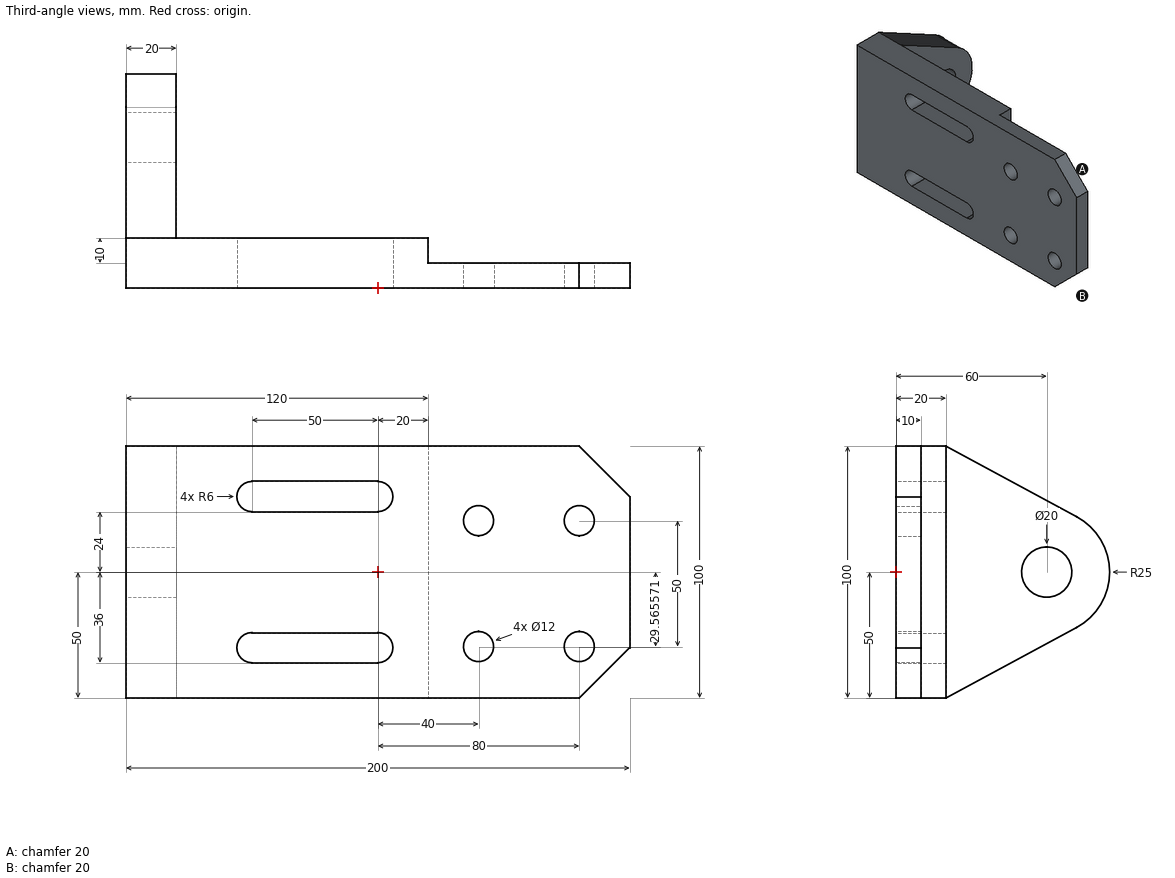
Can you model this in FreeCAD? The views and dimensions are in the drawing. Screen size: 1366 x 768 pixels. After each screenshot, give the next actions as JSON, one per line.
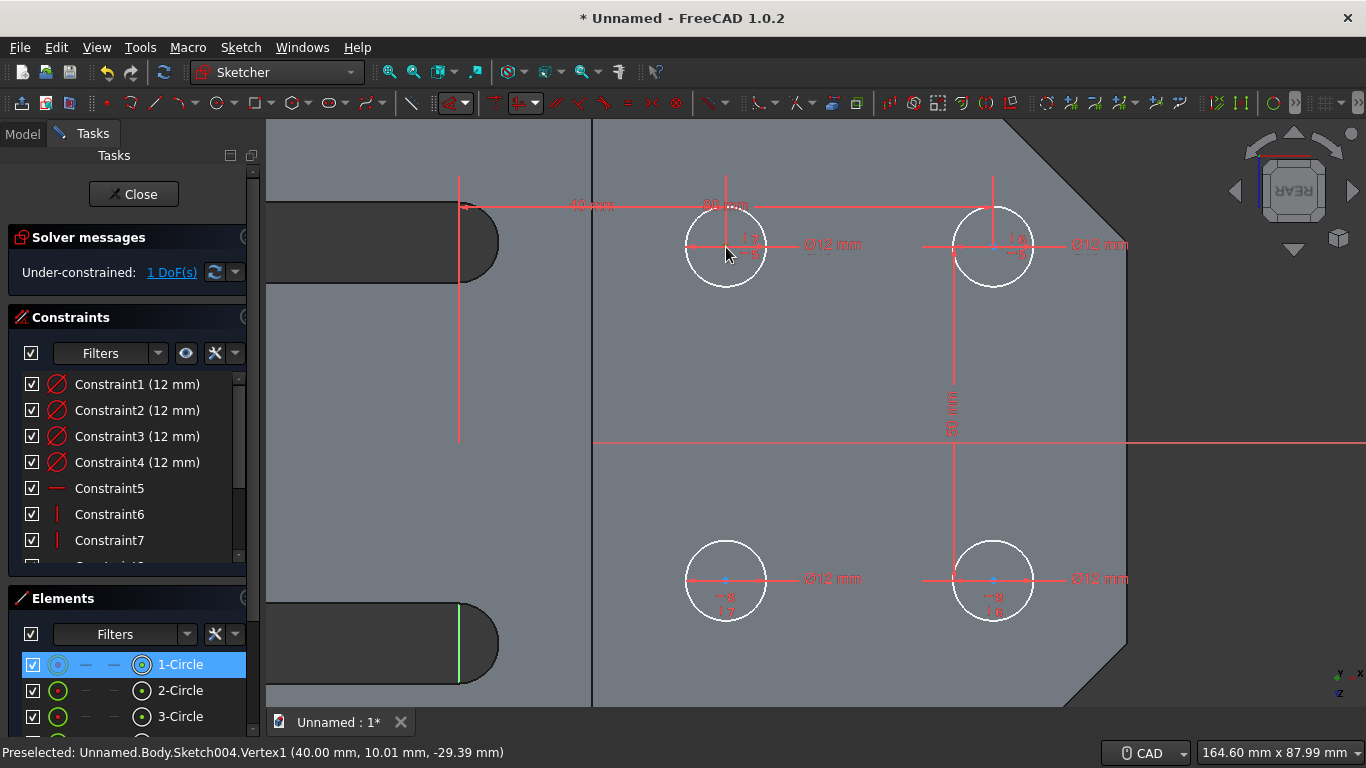
{"action": "key", "text": "i"}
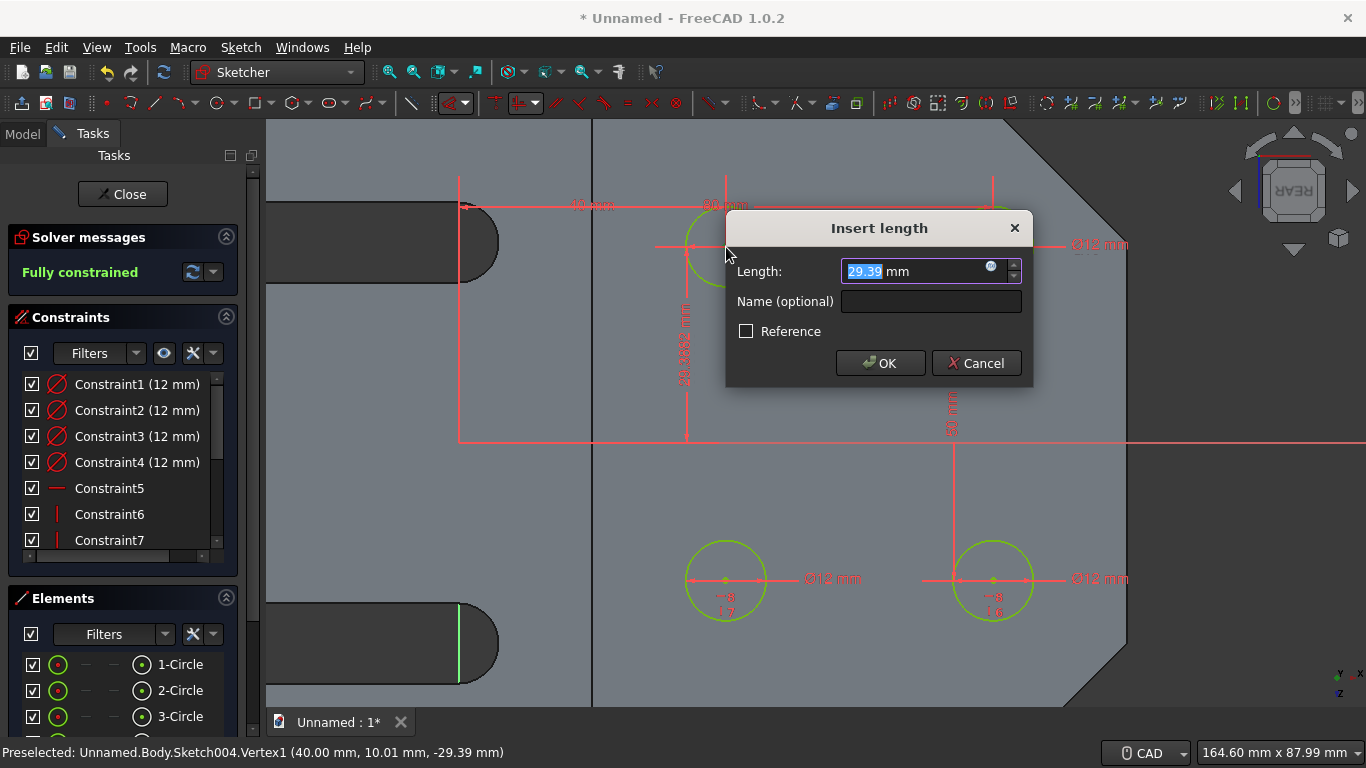
{"action": "type", "text": "29.565571"}
{"action": "key", "text": "Return"}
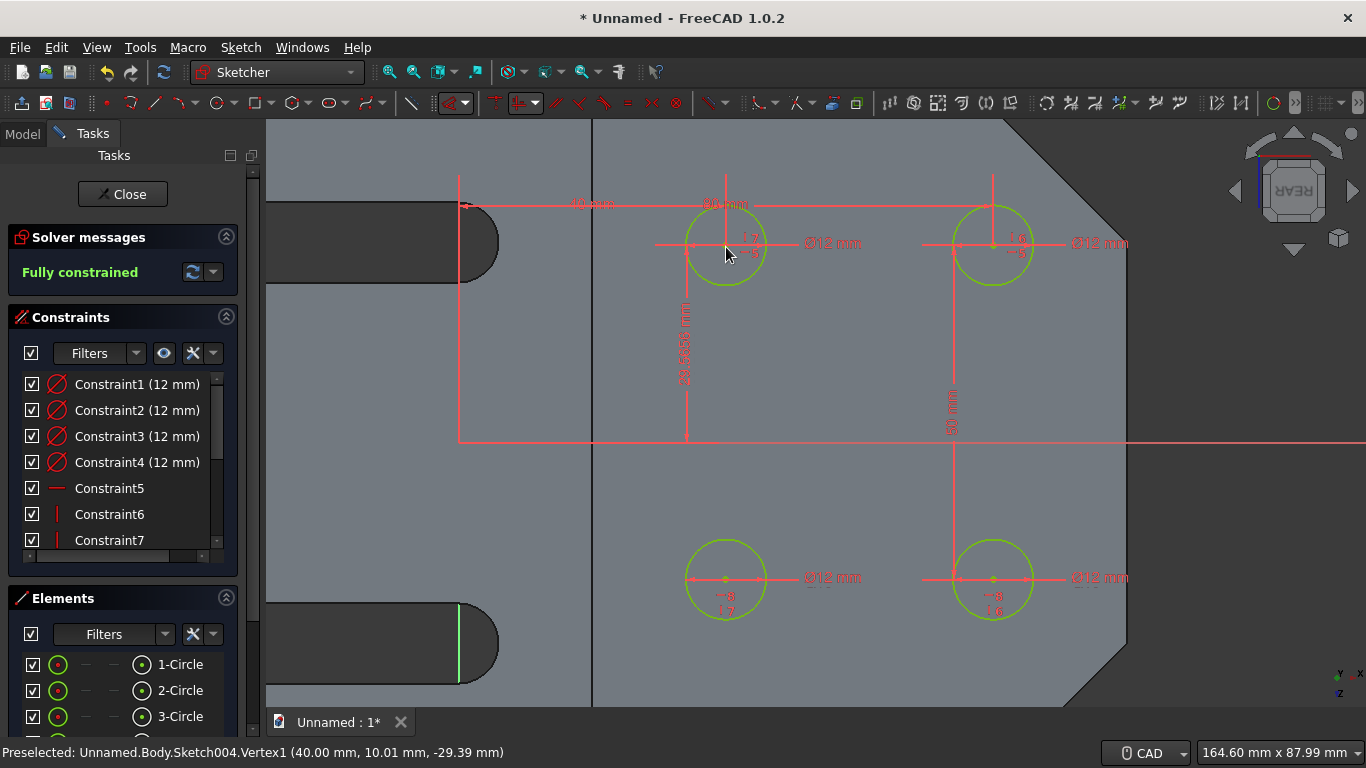
{"action": "left_click", "coordinate": [123, 194]}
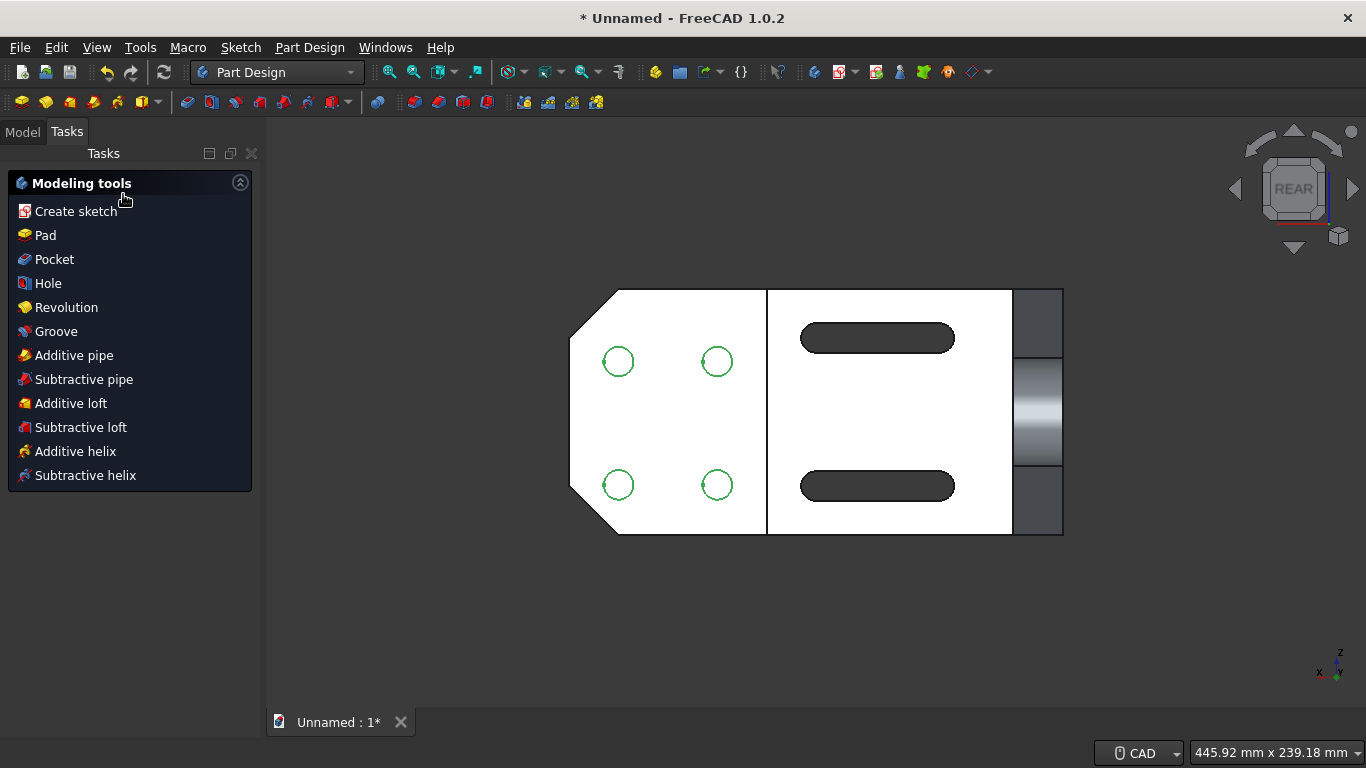
{"action": "left_click", "coordinate": [188, 102]}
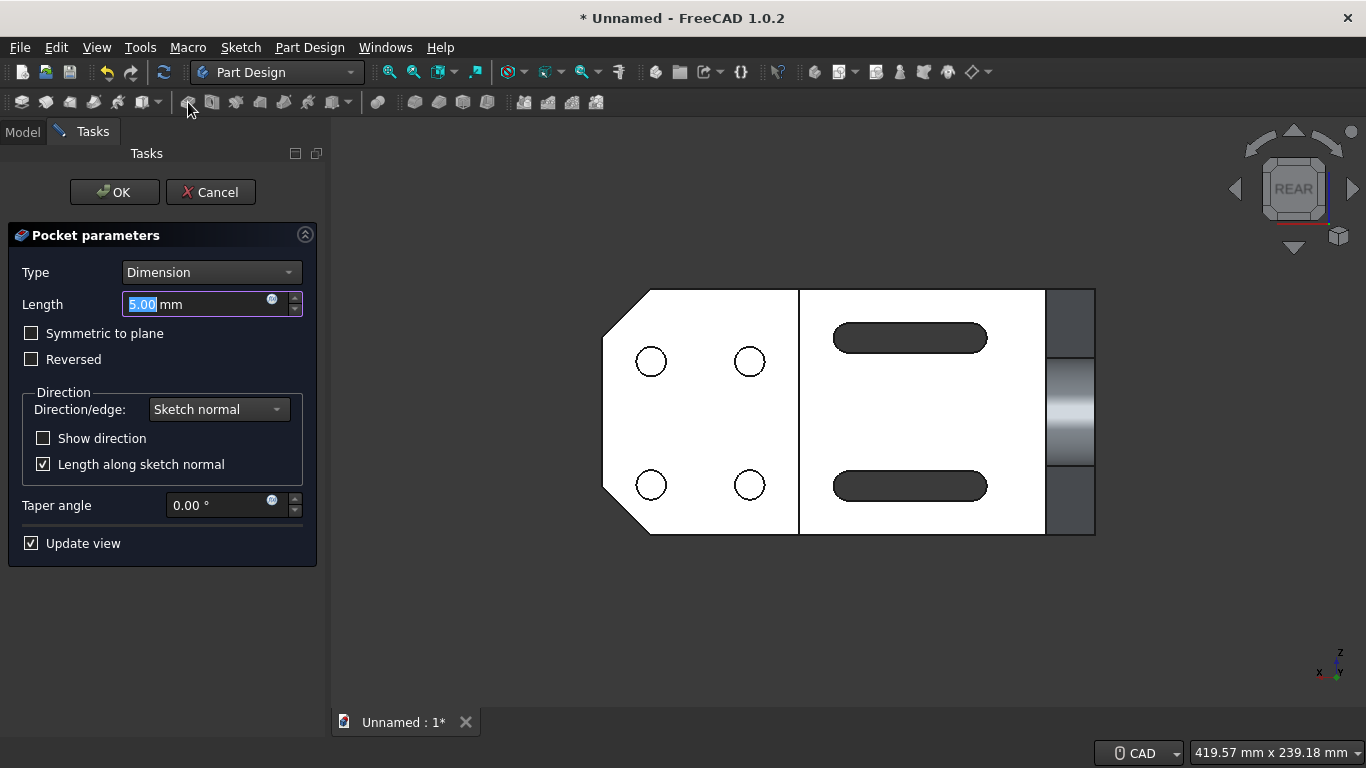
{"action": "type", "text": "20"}
{"action": "key", "text": "Tab"}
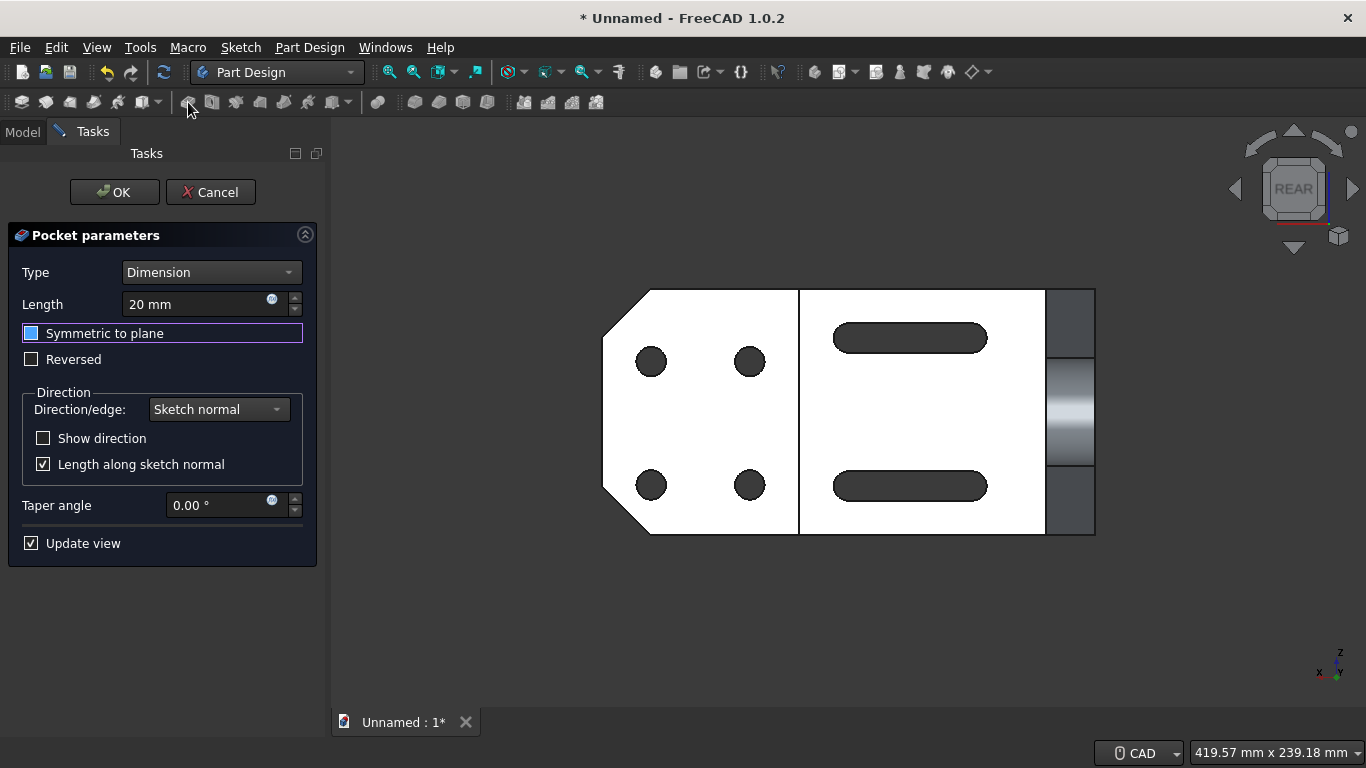
{"action": "left_click", "coordinate": [115, 192]}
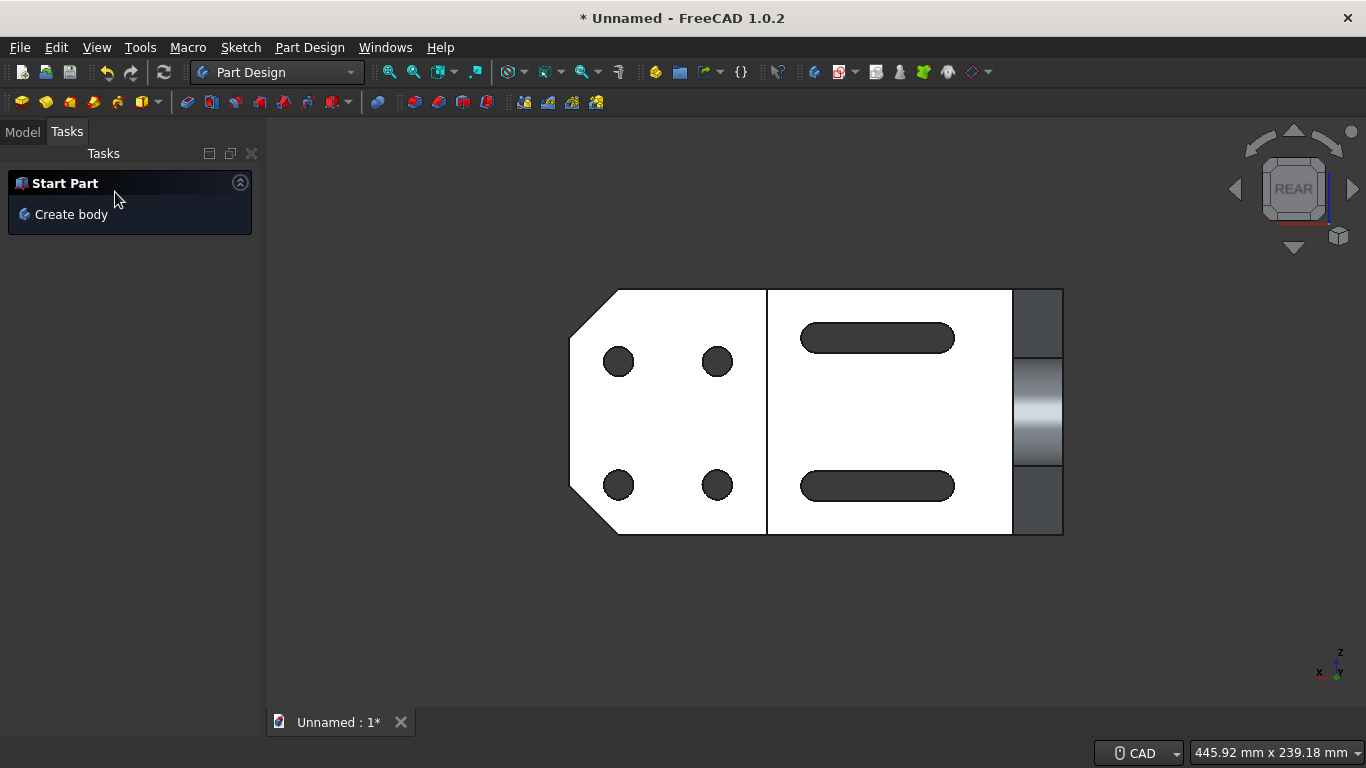
{"action": "key", "text": "0"}